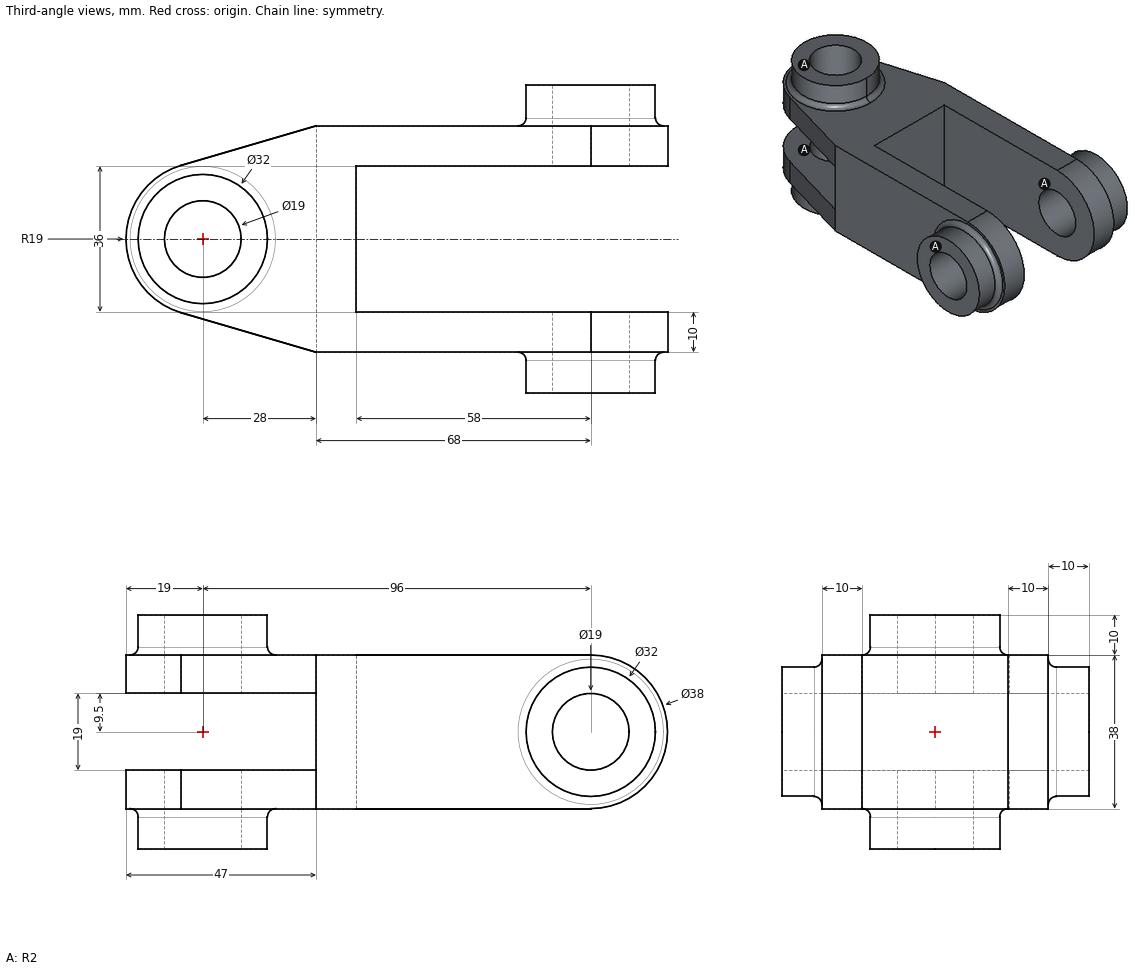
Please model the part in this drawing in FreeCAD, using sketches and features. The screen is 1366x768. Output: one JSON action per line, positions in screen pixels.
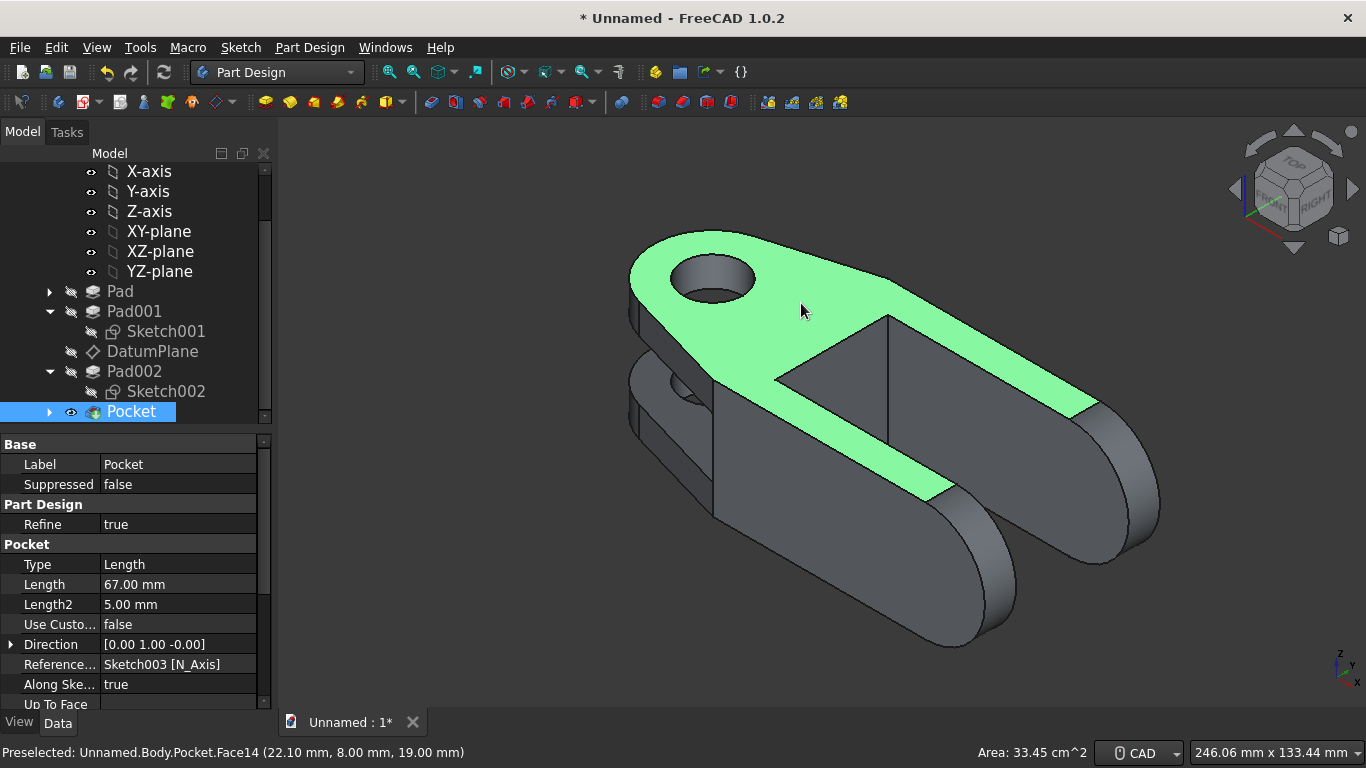
{"action": "left_click", "coordinate": [84, 102]}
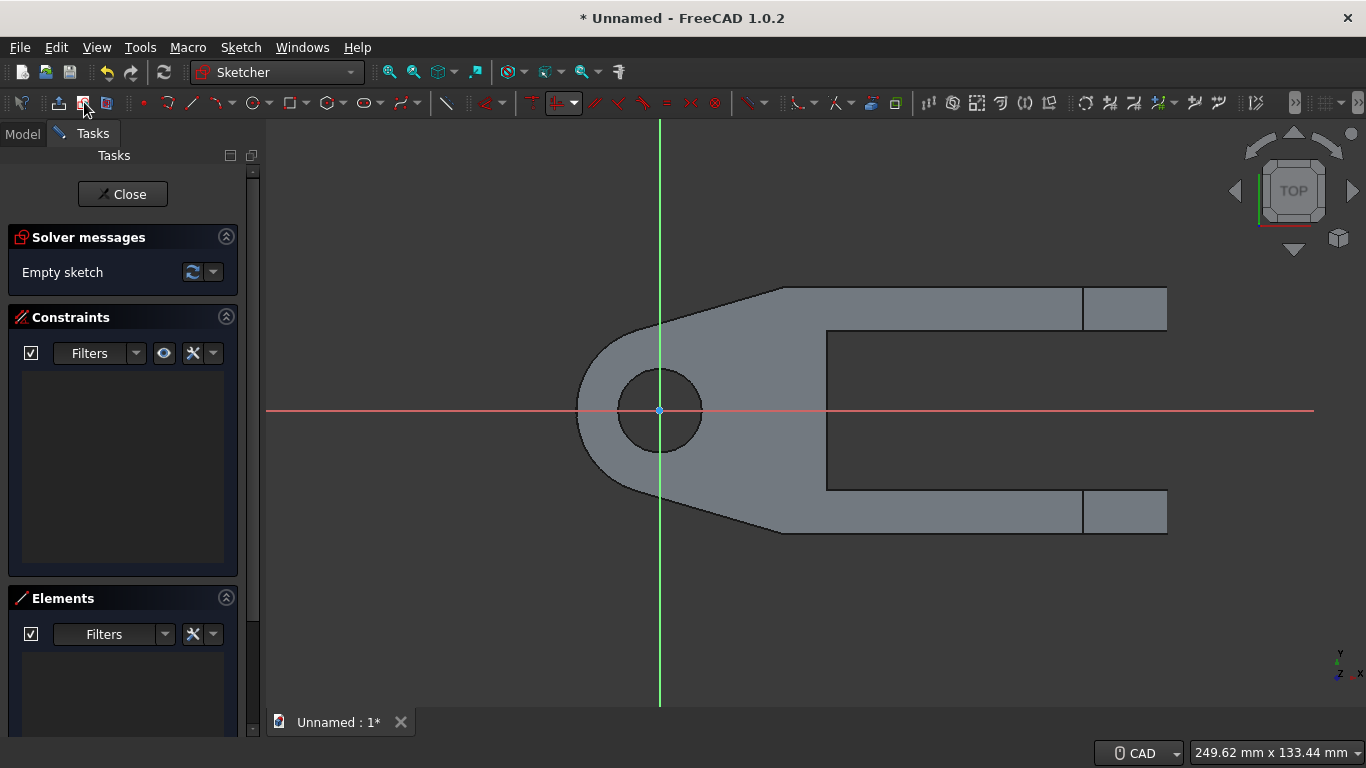
{"action": "scroll", "coordinate": [609, 409], "scroll_direction": "up", "scroll_amount": 5}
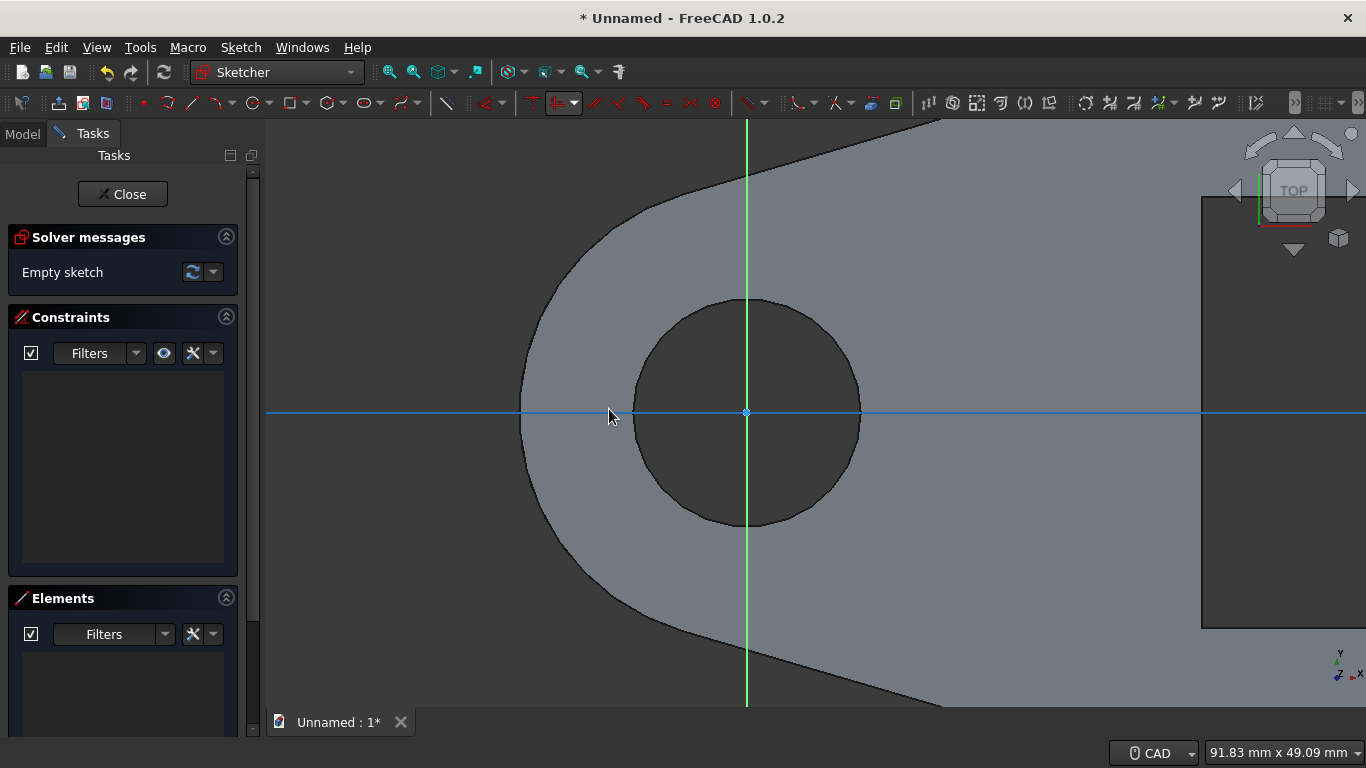
{"action": "left_click", "coordinate": [254, 104]}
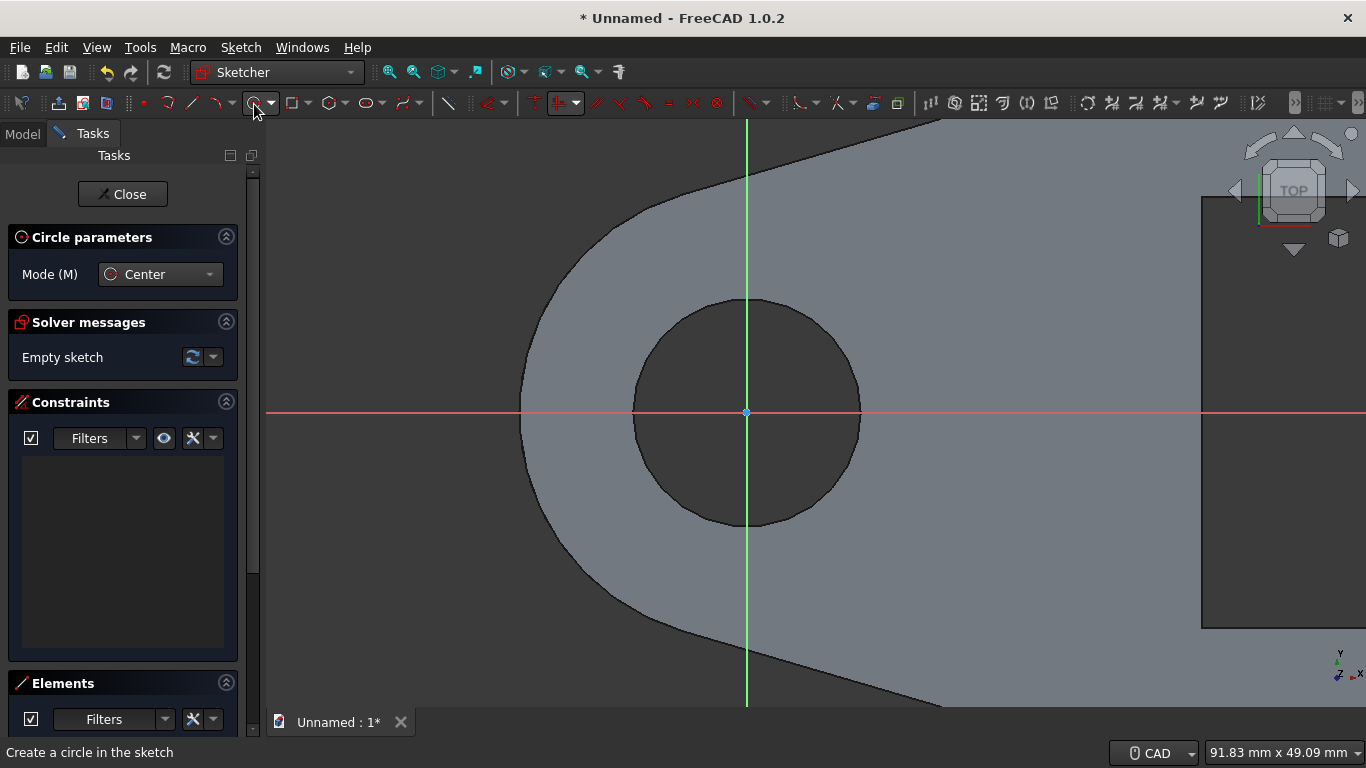
{"action": "left_click", "coordinate": [747, 413]}
{"action": "left_click", "coordinate": [882, 277]}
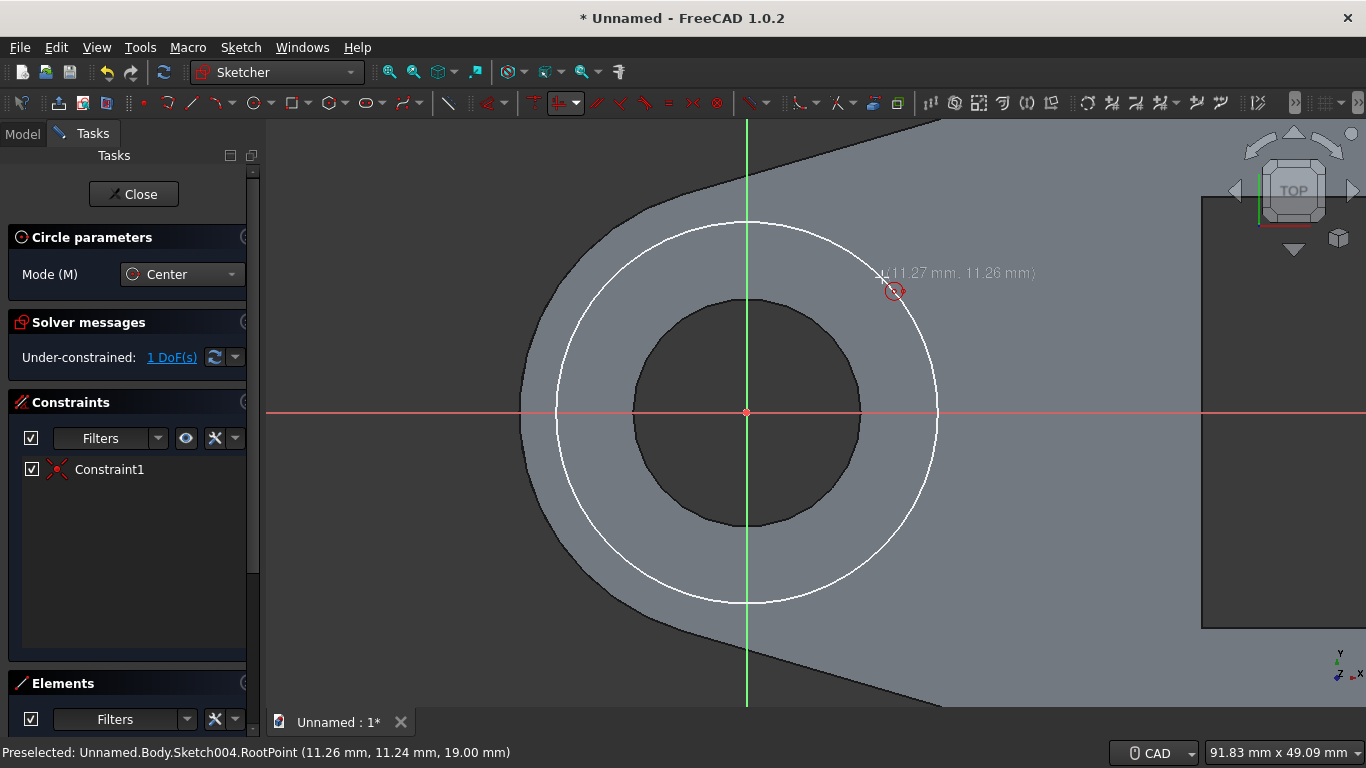
{"action": "left_click", "coordinate": [747, 413]}
{"action": "left_click", "coordinate": [827, 332]}
{"action": "key", "text": "Escape"}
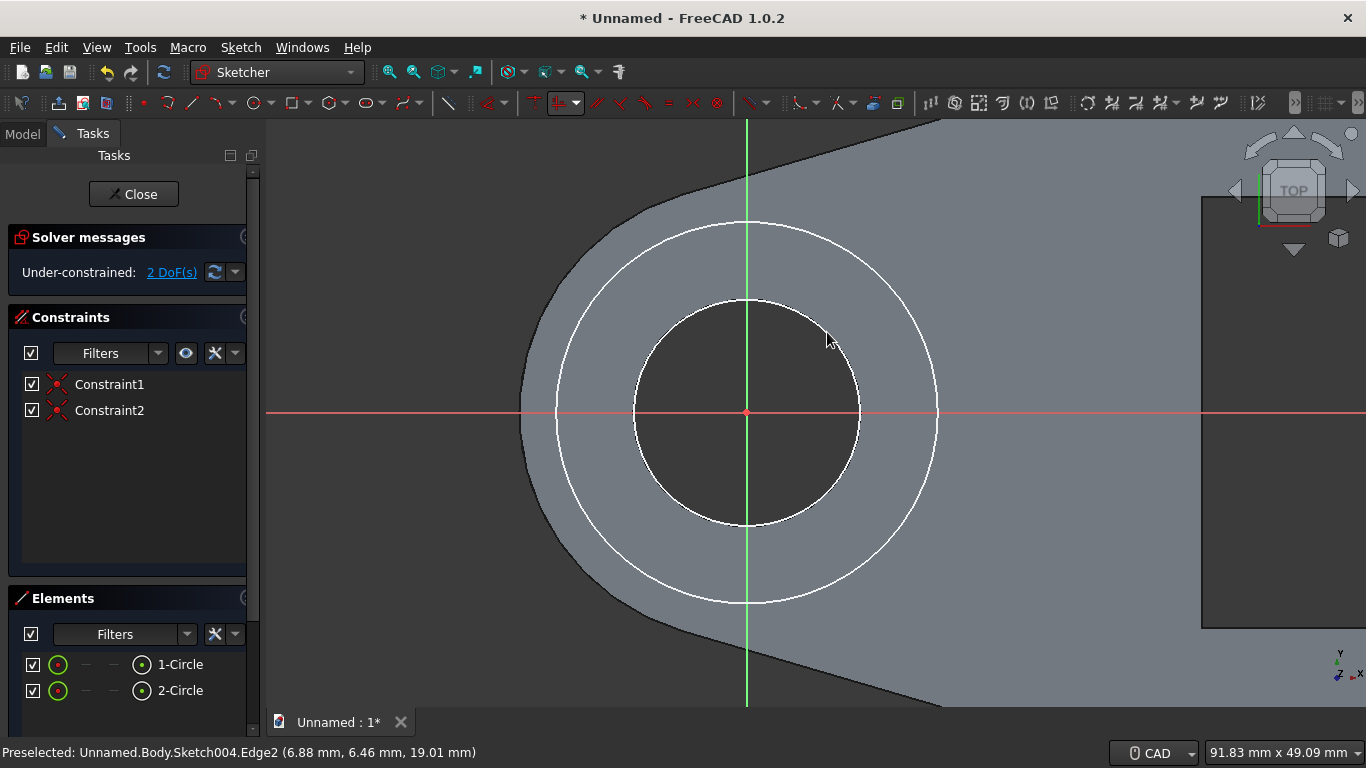
{"action": "key", "text": "d"}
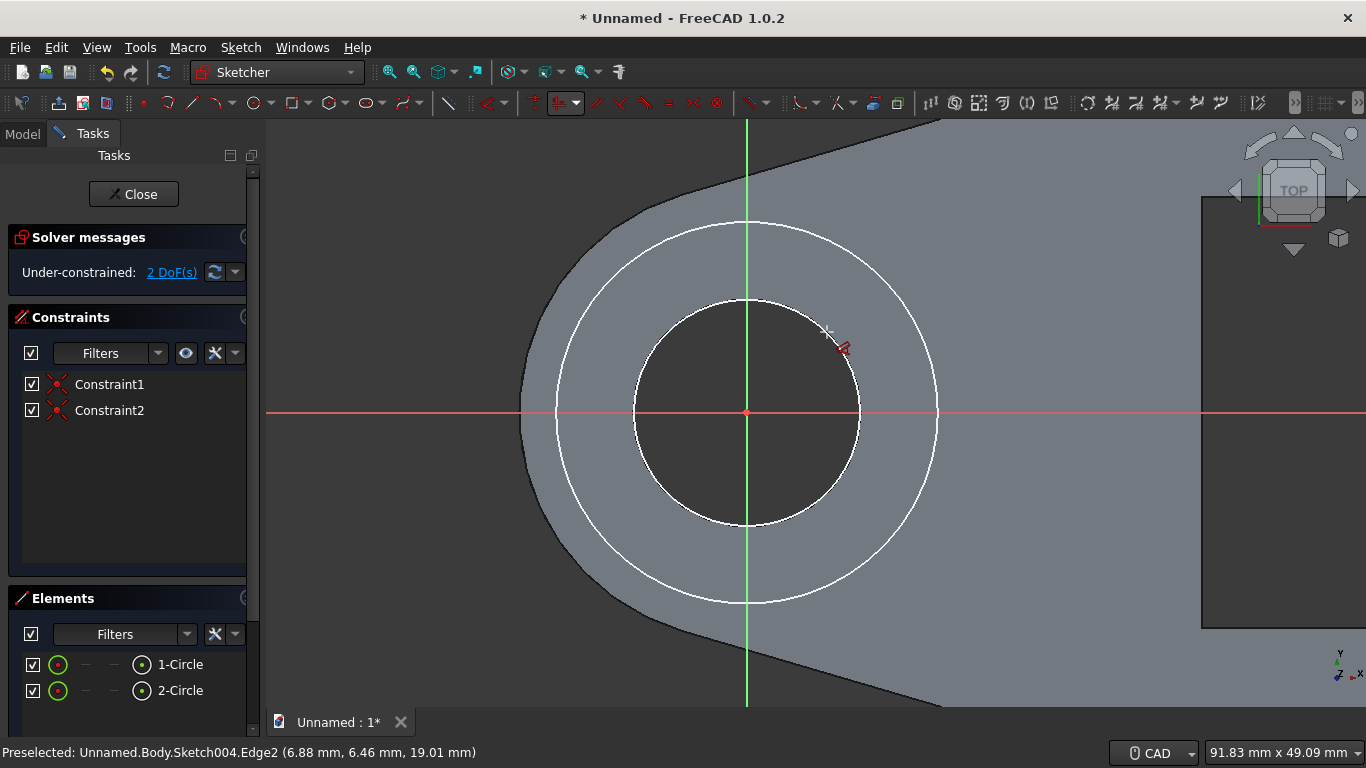
{"action": "left_click", "coordinate": [882, 278]}
{"action": "left_click", "coordinate": [905, 255]}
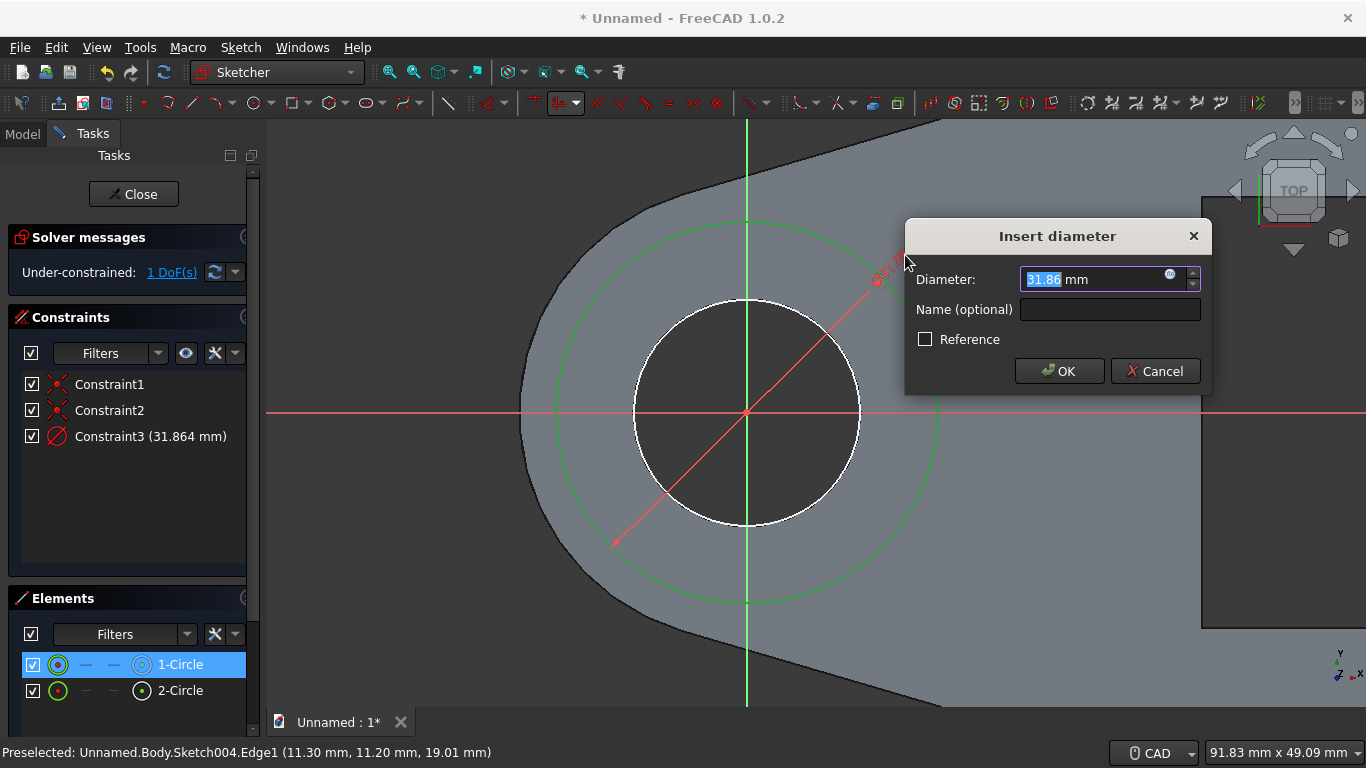
{"action": "type", "text": "32"}
{"action": "key", "text": "Return"}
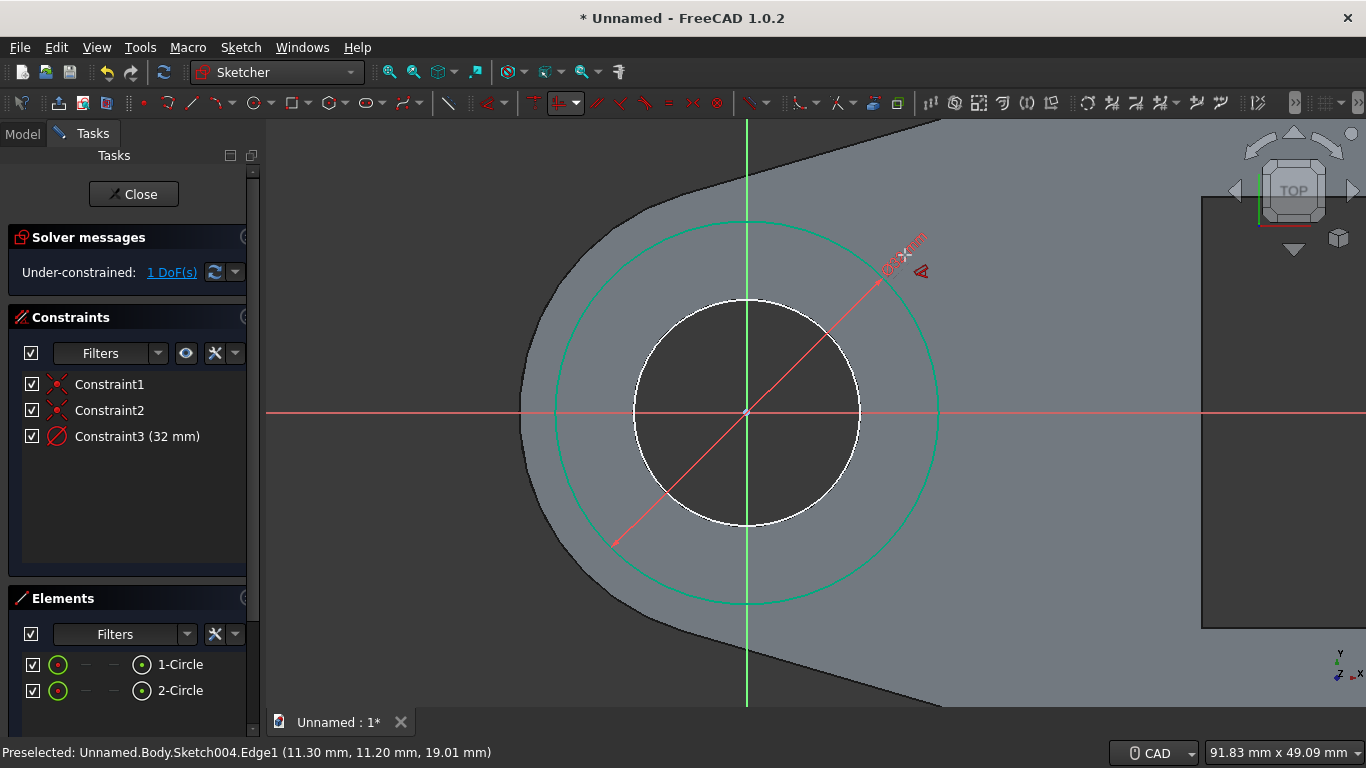
{"action": "left_click", "coordinate": [827, 333]}
{"action": "left_click", "coordinate": [850, 310]}